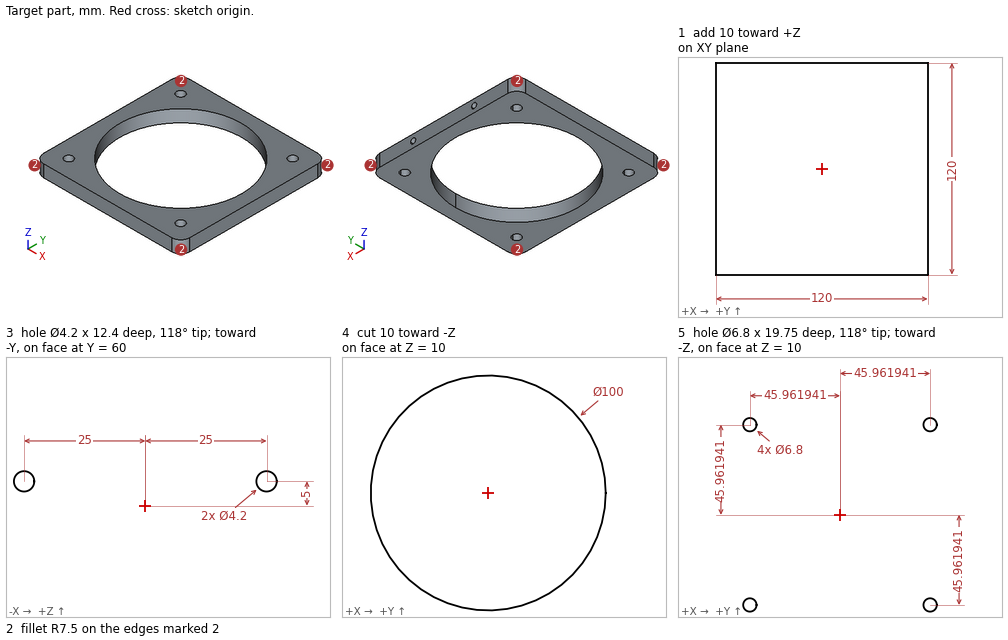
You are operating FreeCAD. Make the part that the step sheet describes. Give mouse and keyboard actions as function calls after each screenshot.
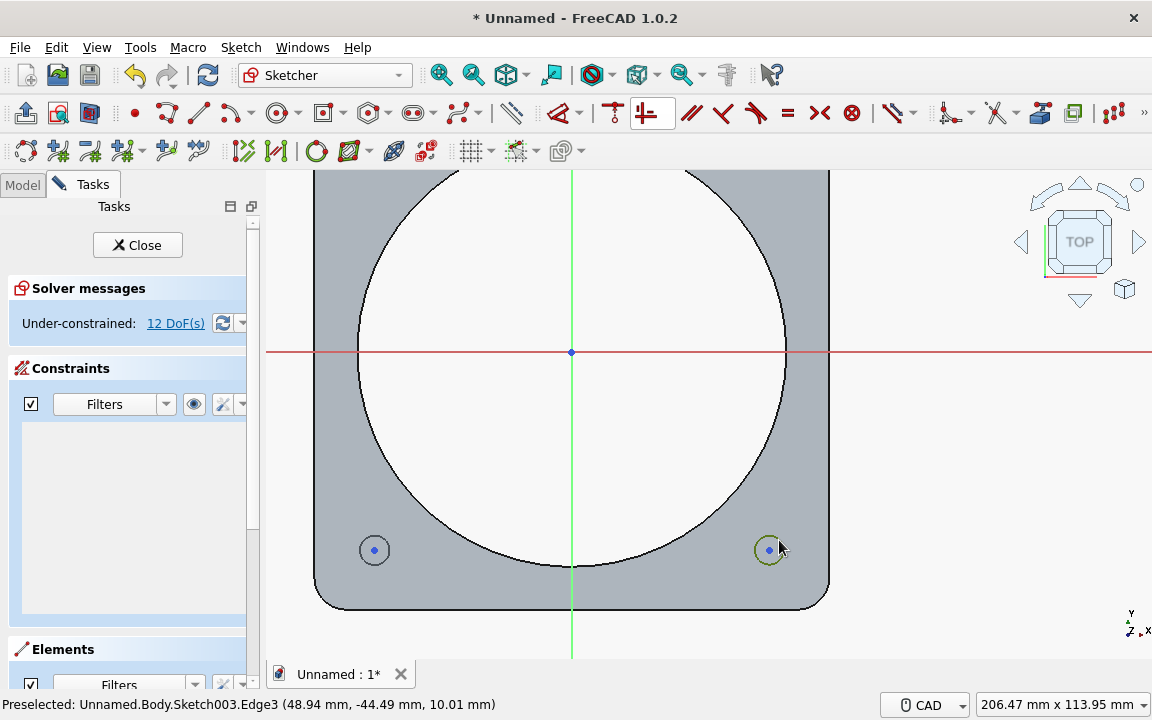
click(385, 540)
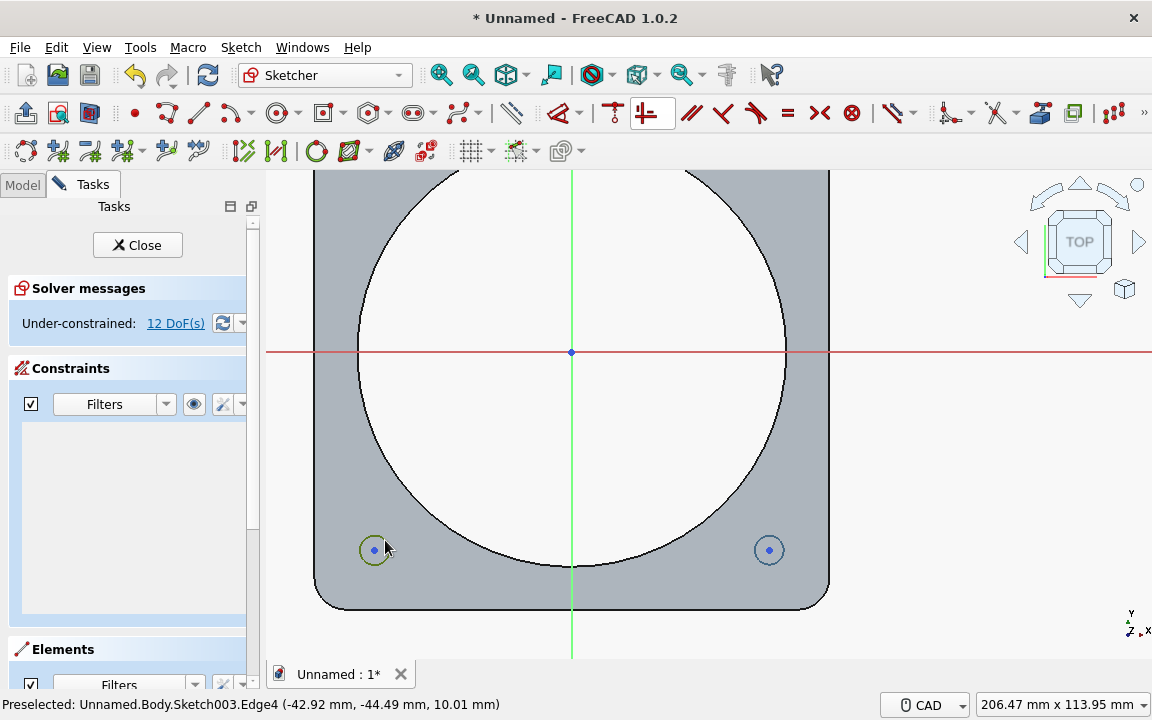
click(788, 114)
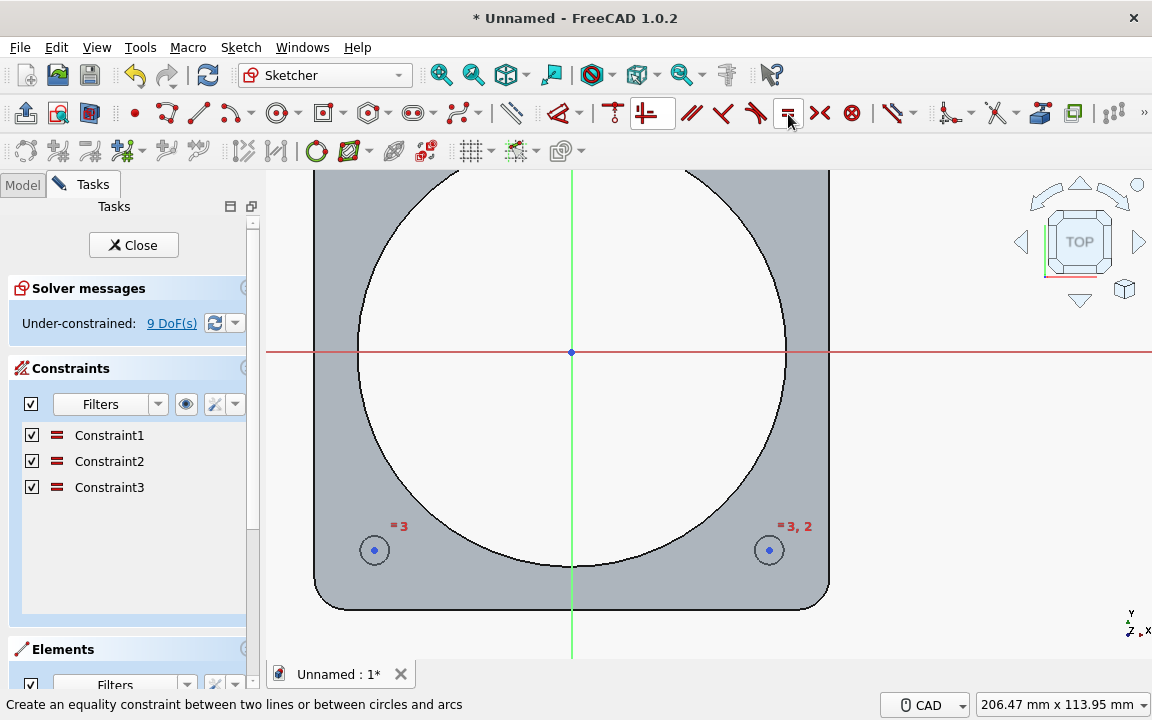
scroll(780, 541, down, 2)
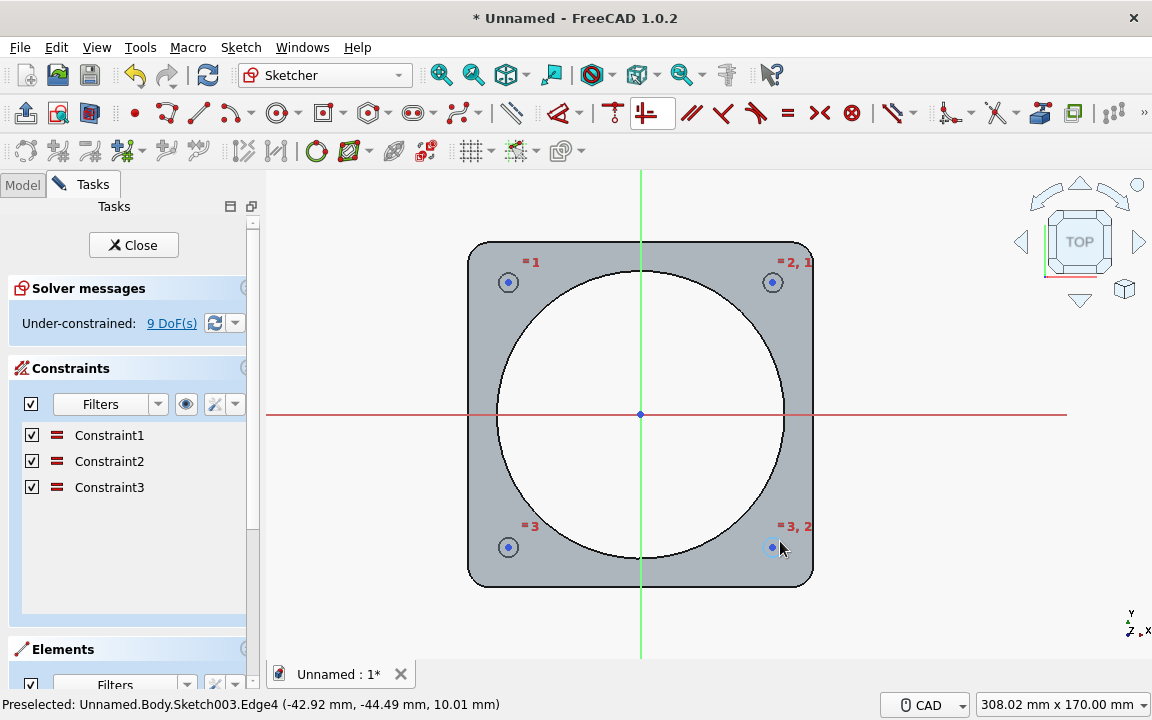
click(509, 283)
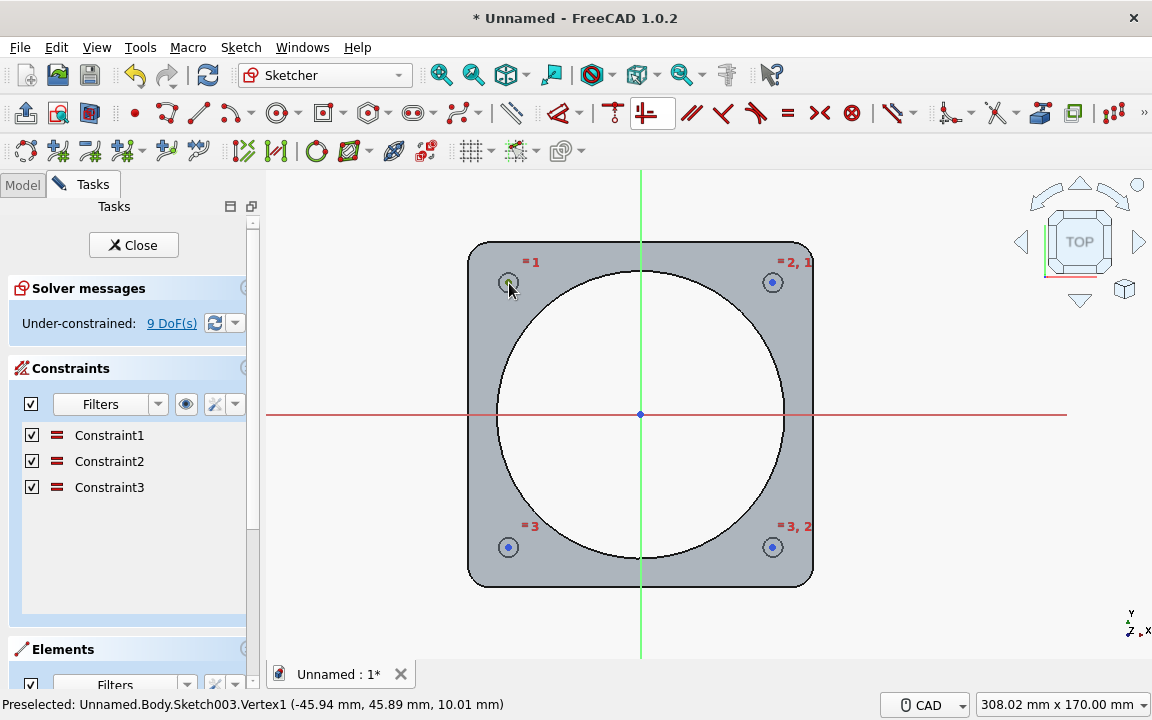
click(773, 283)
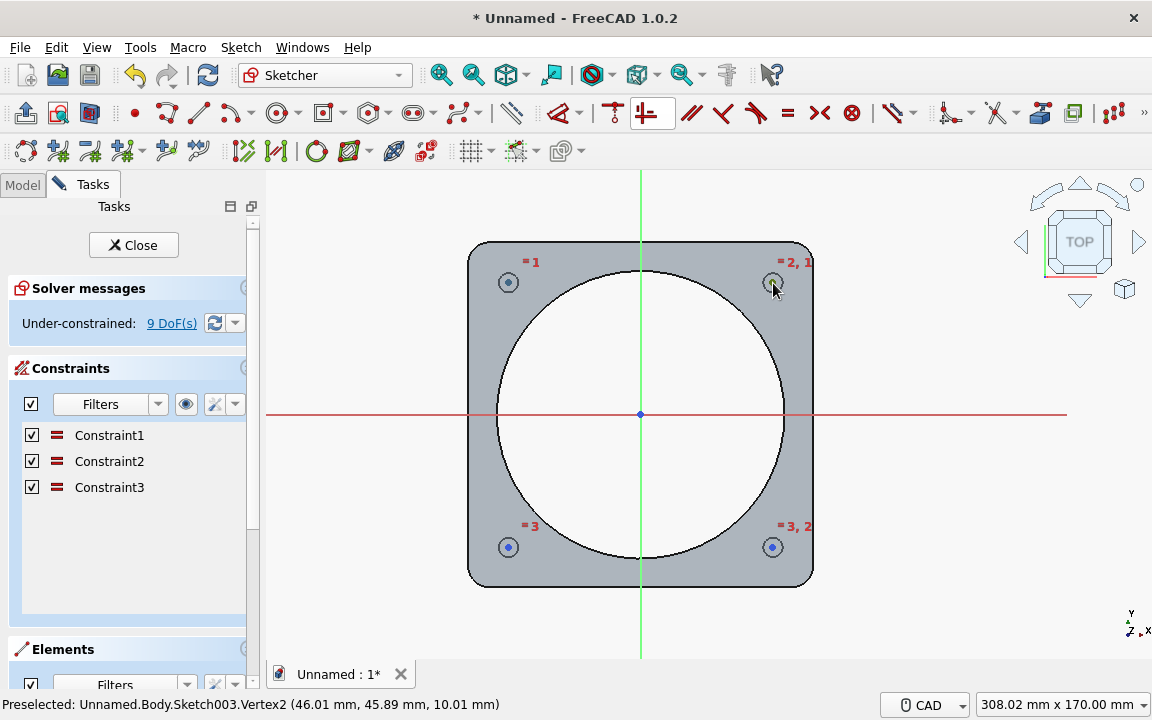
key(h)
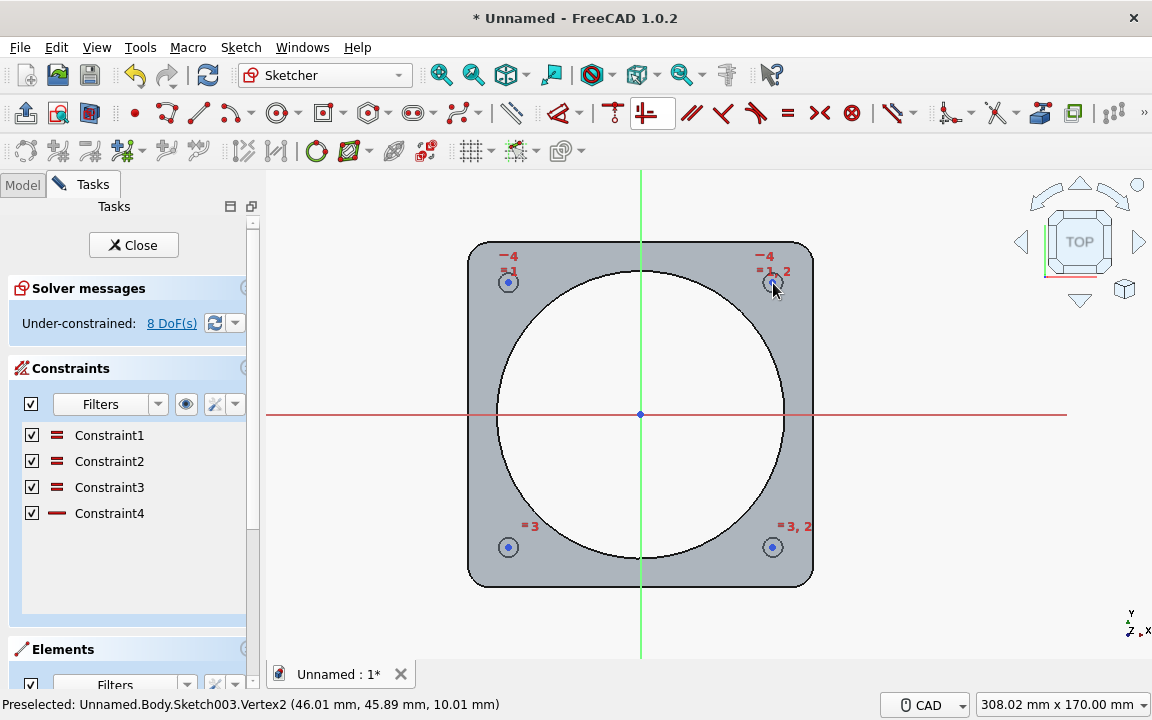
click(773, 283)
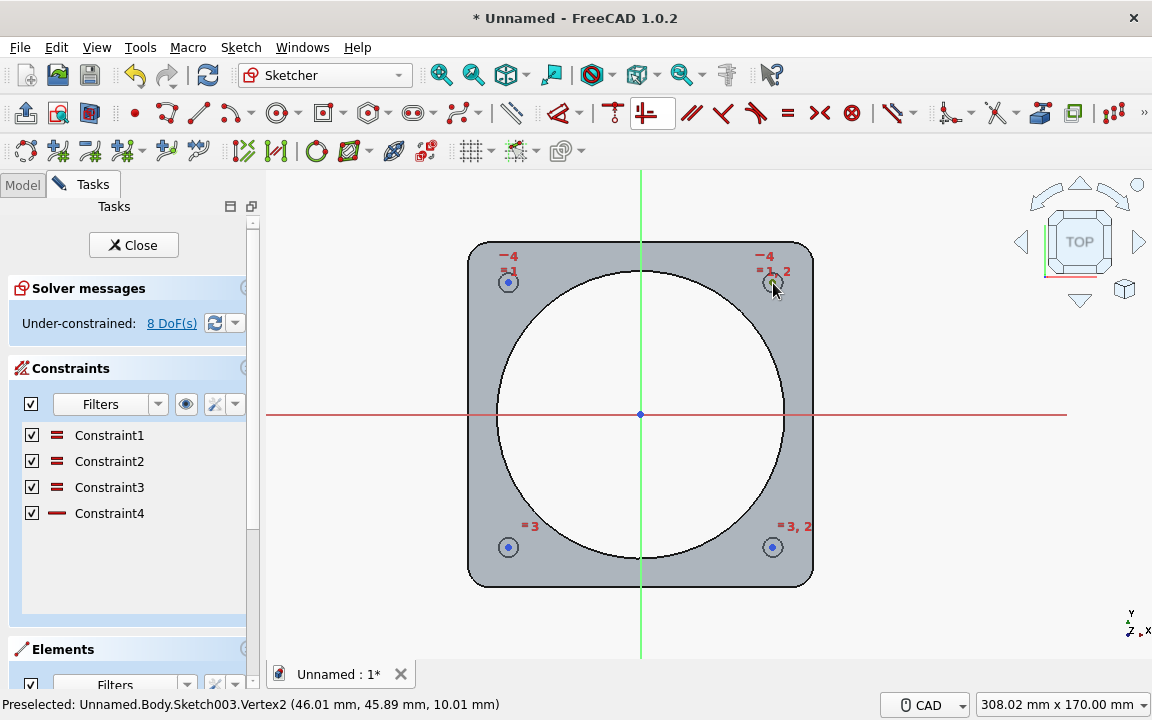
click(773, 547)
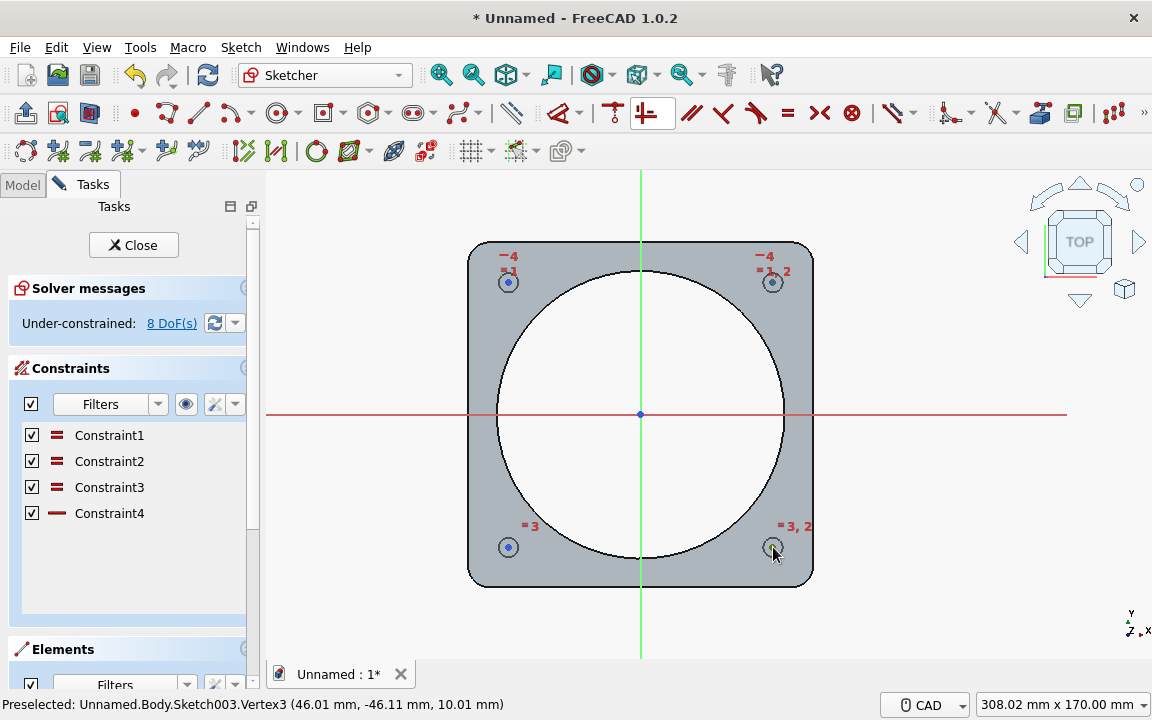
click(670, 114)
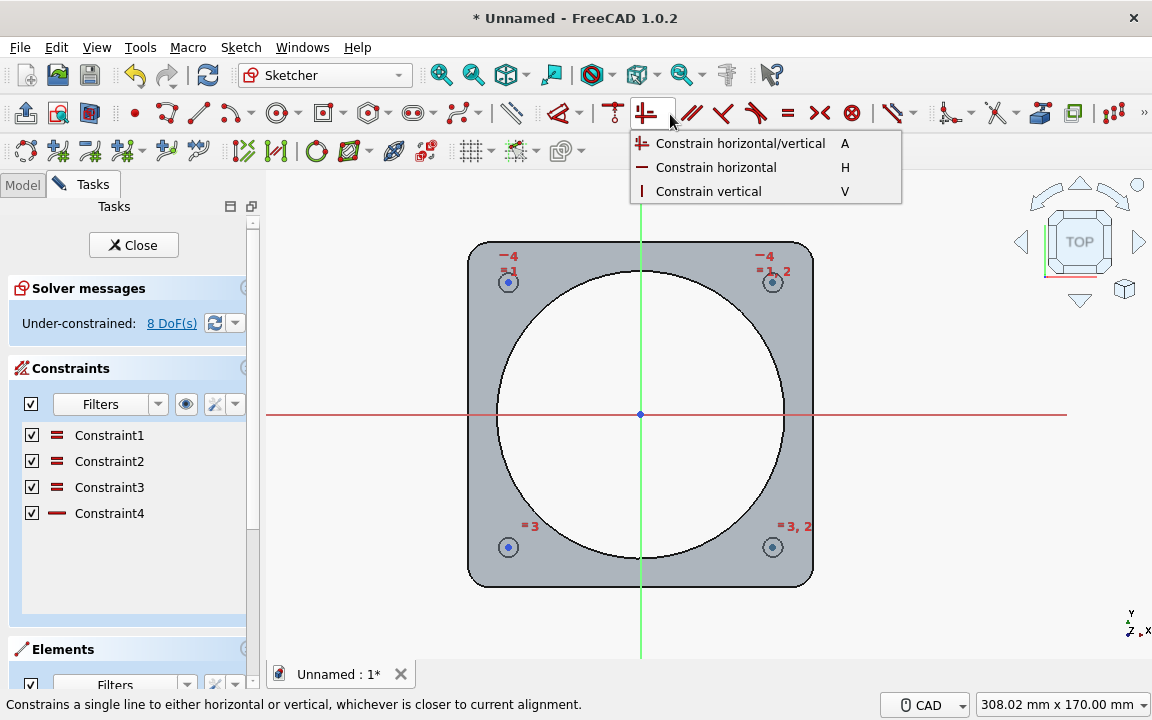
click(766, 191)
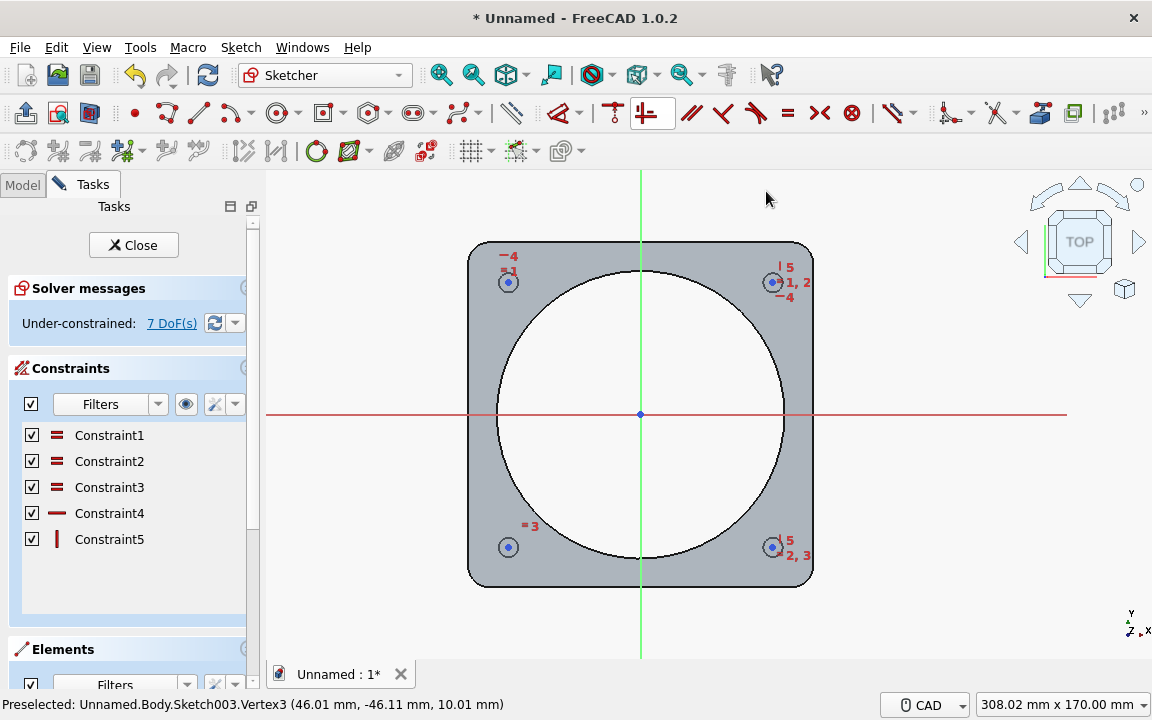
click(509, 283)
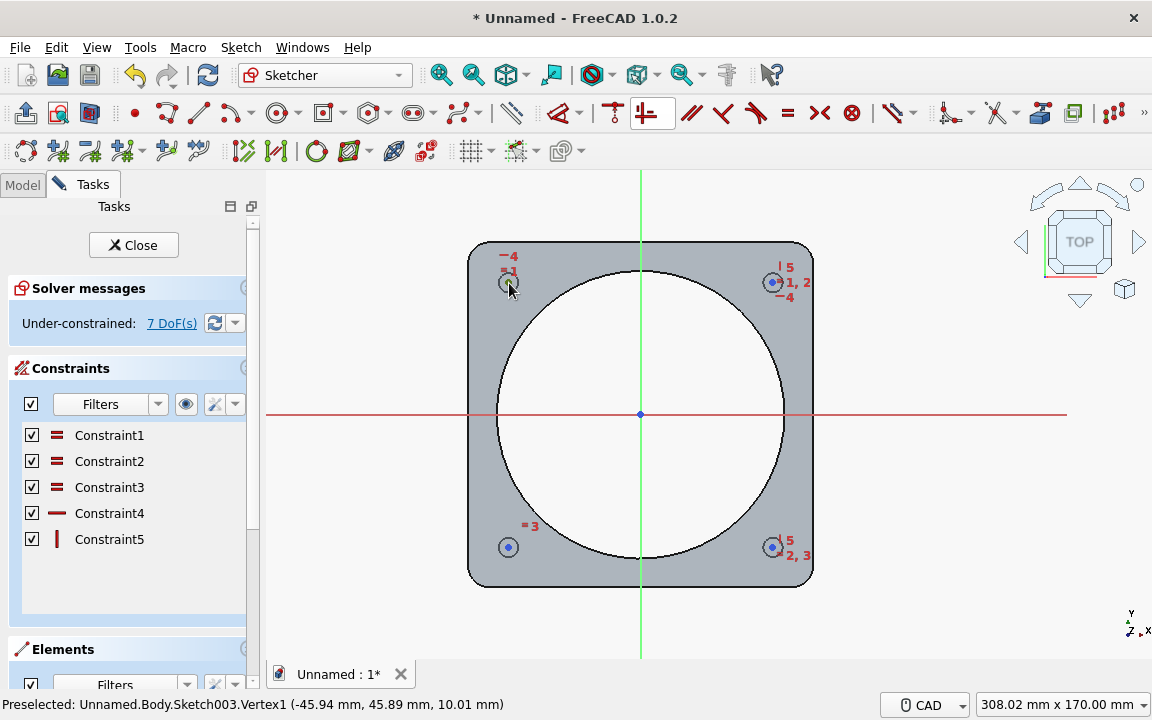
click(509, 548)